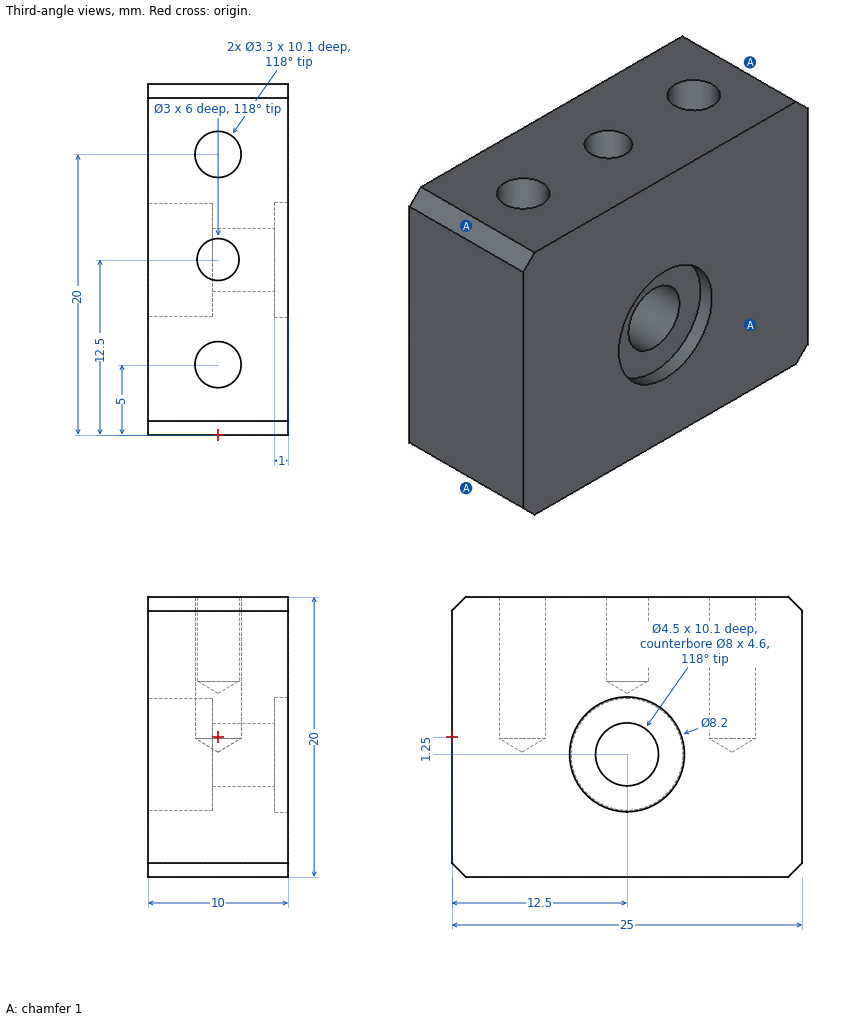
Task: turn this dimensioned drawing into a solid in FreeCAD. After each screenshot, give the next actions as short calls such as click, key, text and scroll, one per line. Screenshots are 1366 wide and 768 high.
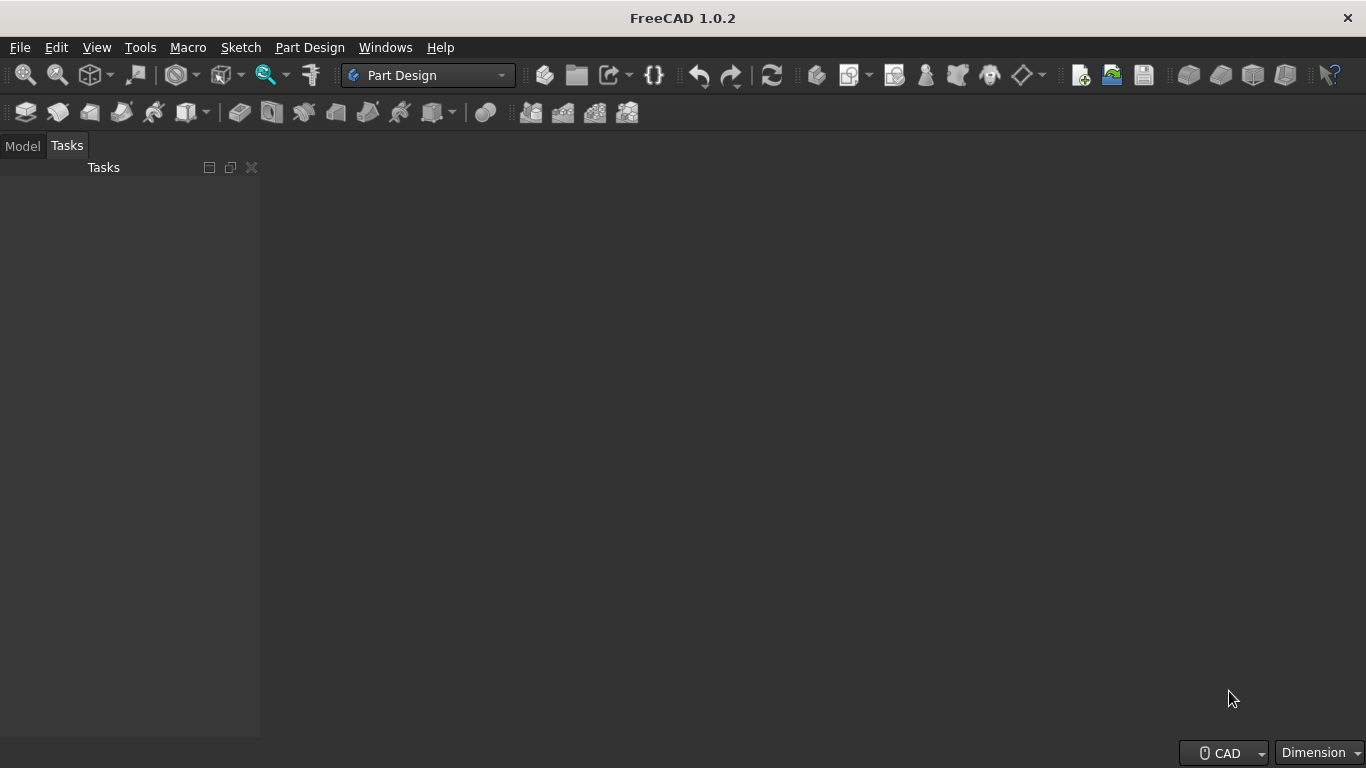
click(1080, 76)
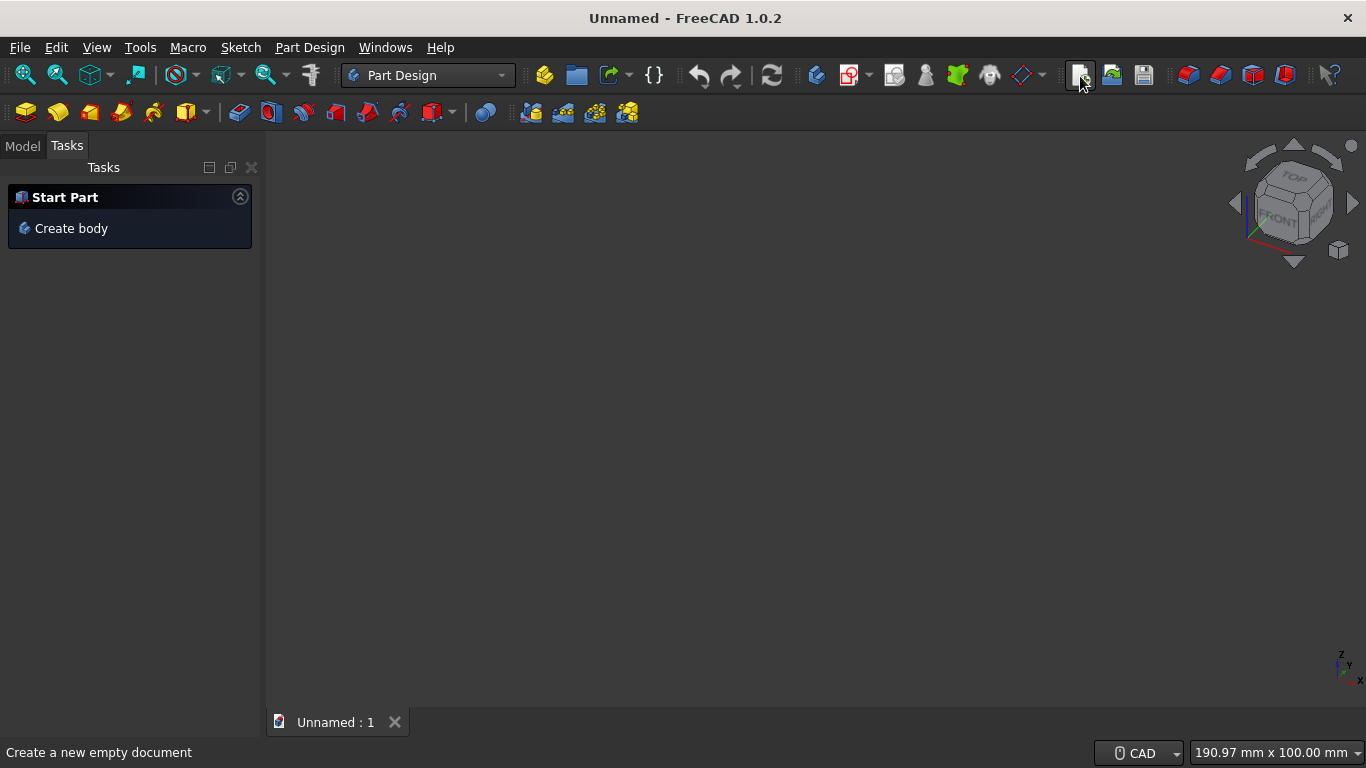
click(850, 76)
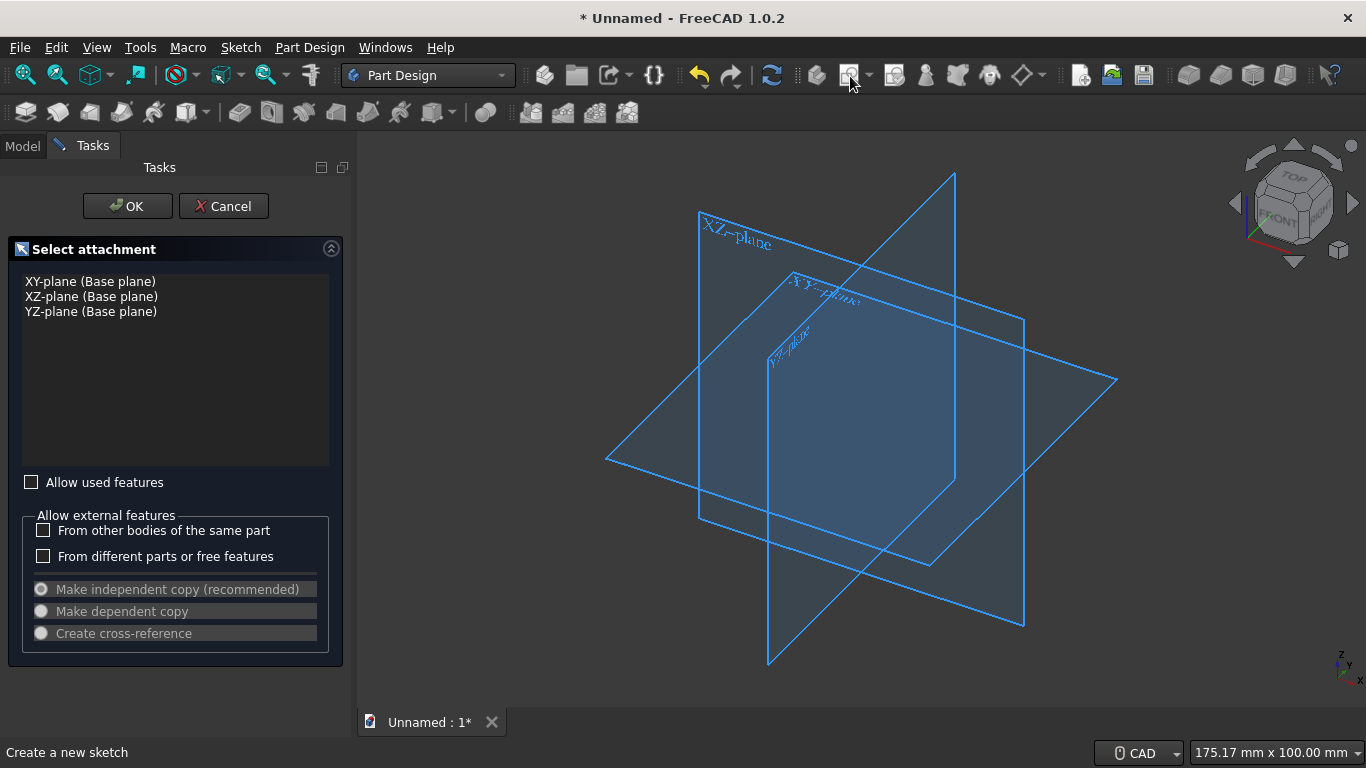
click(82, 296)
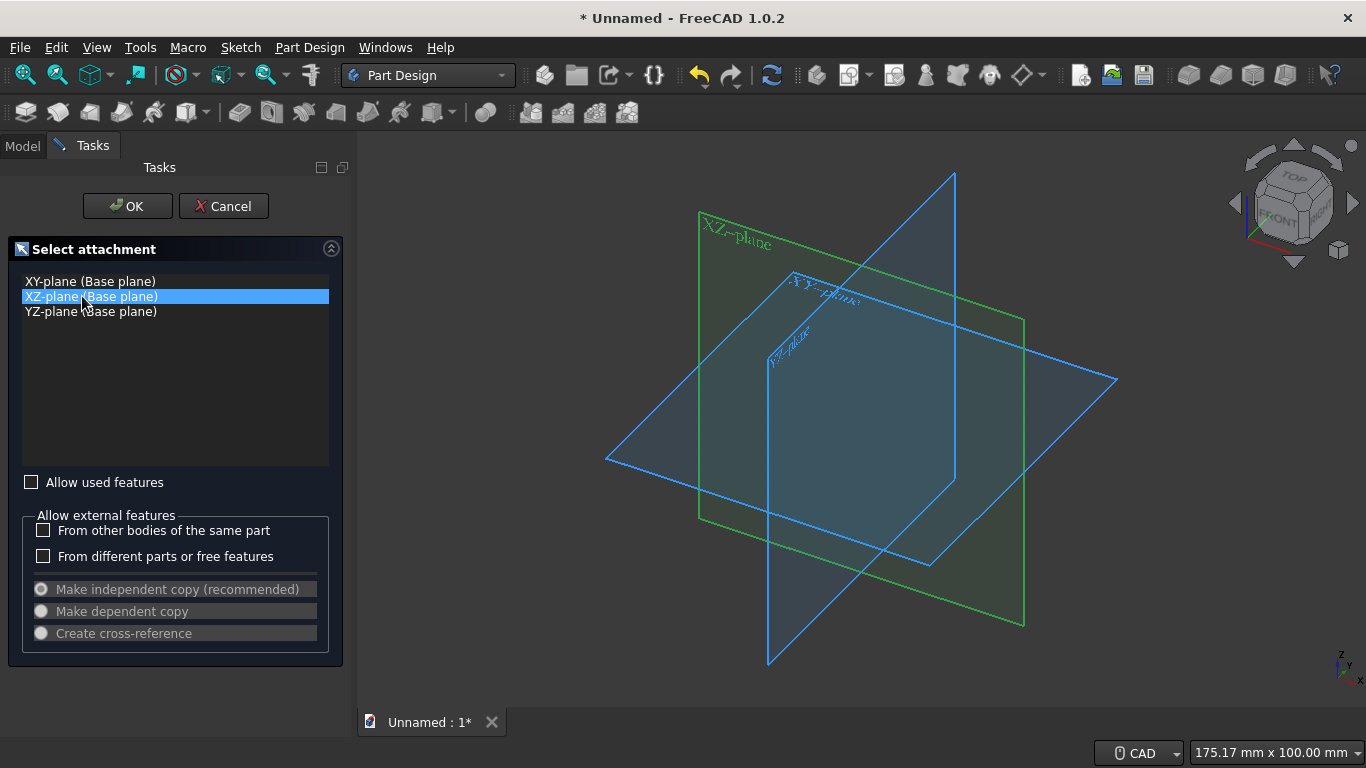
click(128, 206)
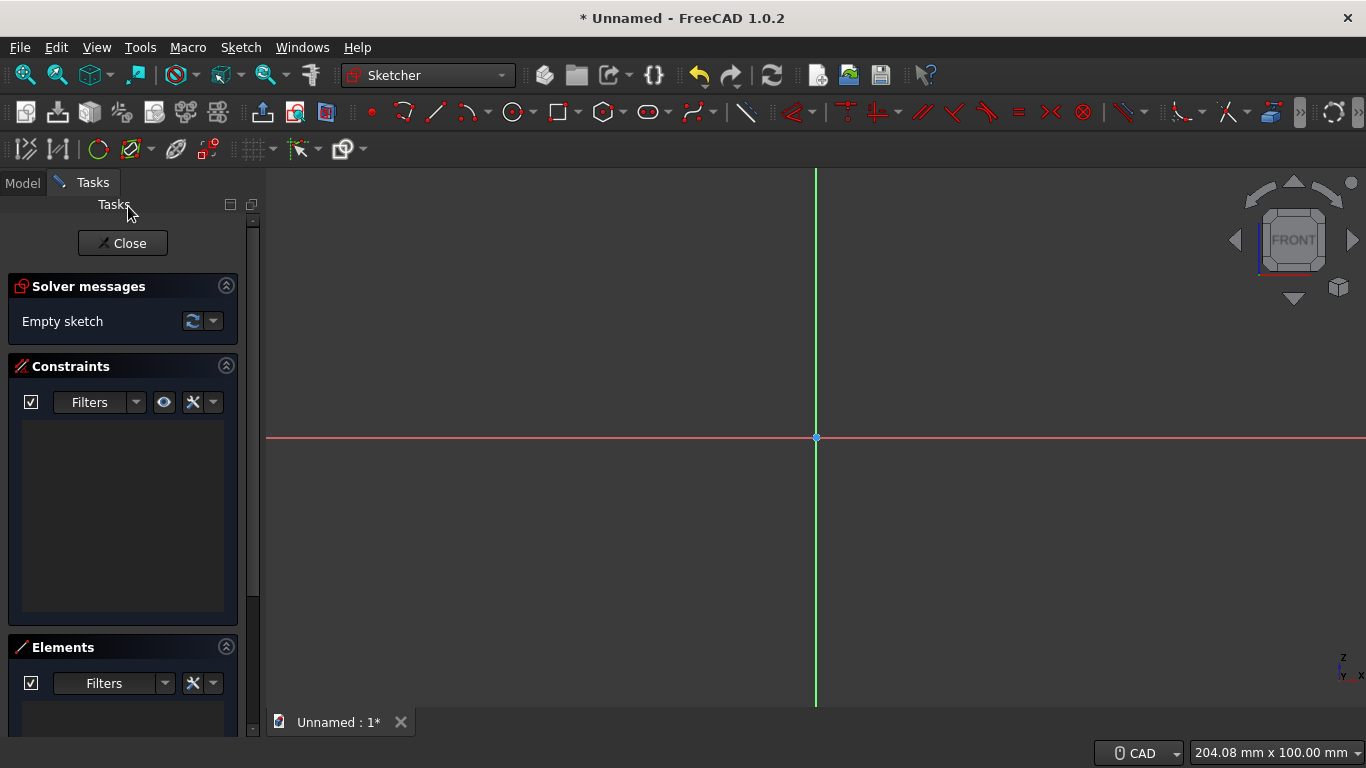
scroll(846, 438, up, 6)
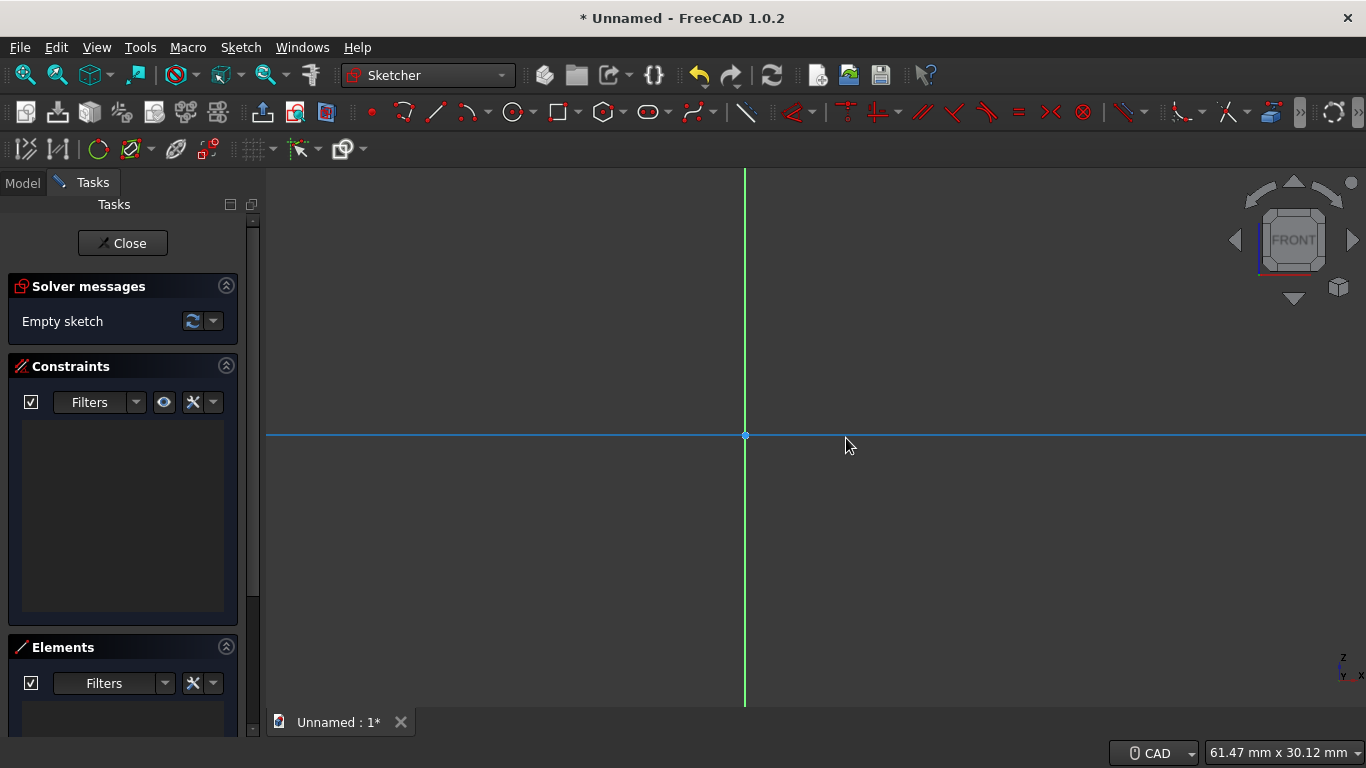
key(g)
key(v)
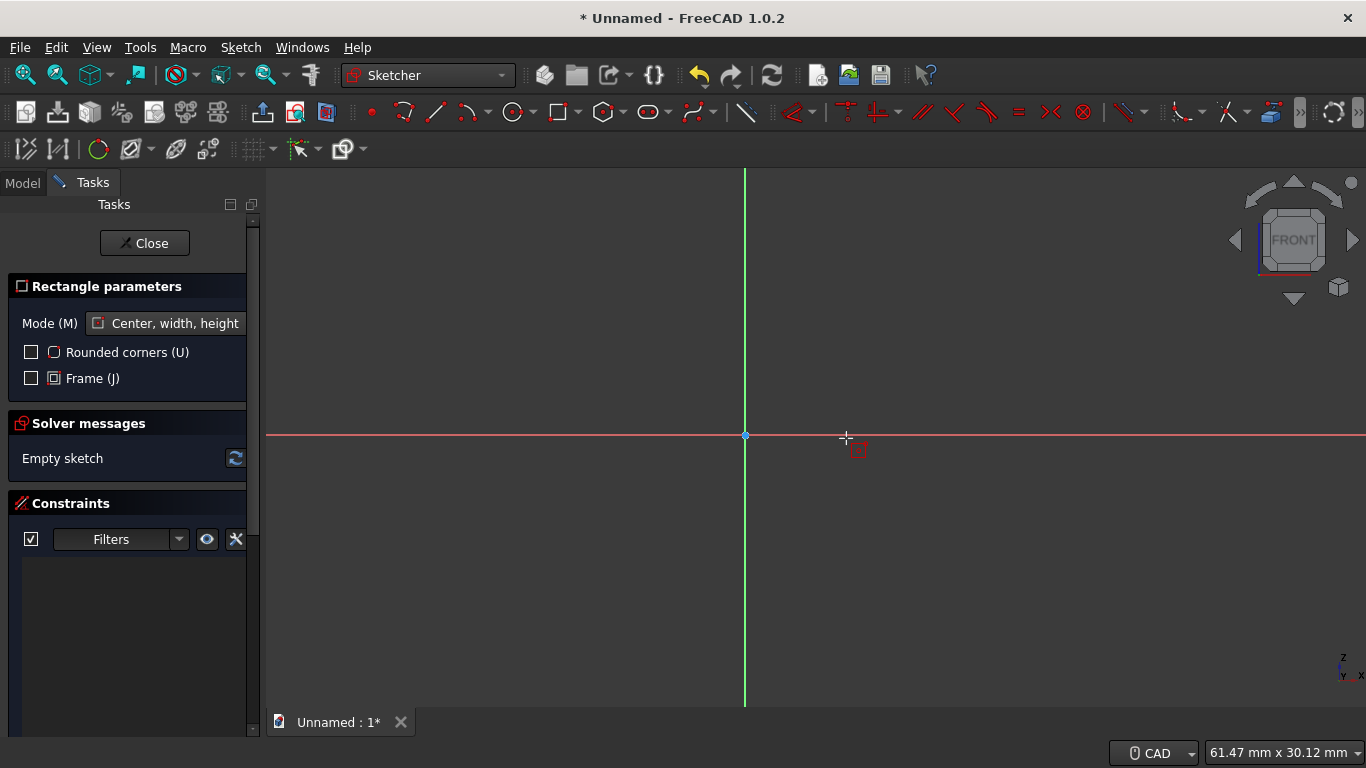
click(745, 435)
click(835, 256)
key(Escape)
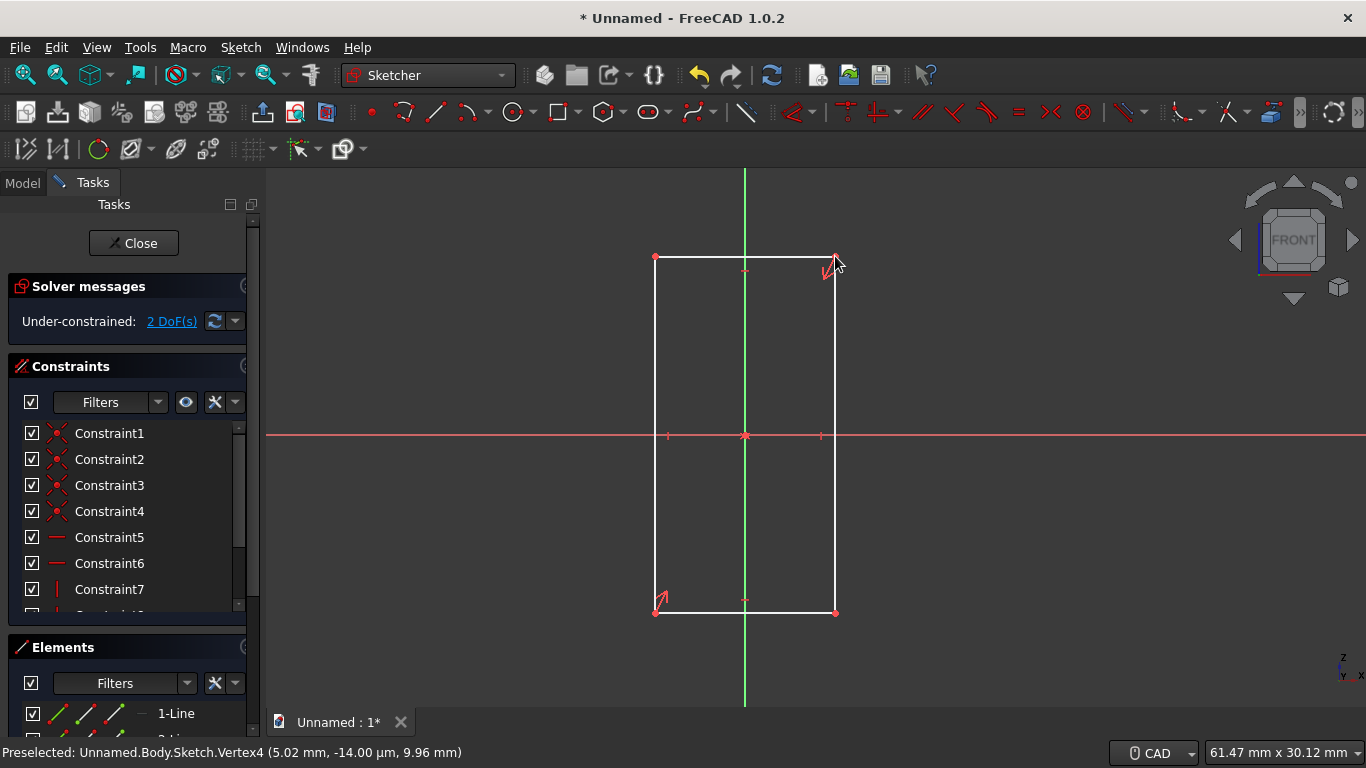
key(d)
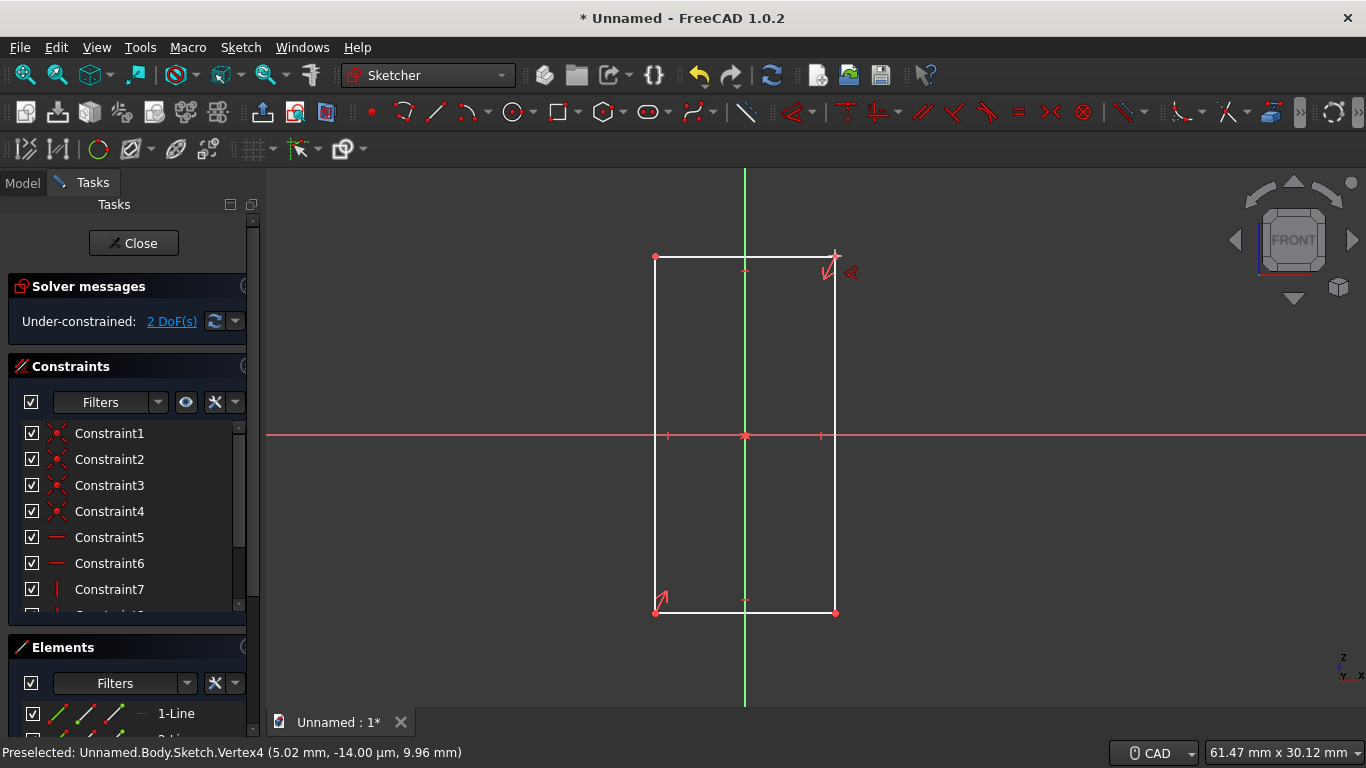
click(709, 613)
click(704, 647)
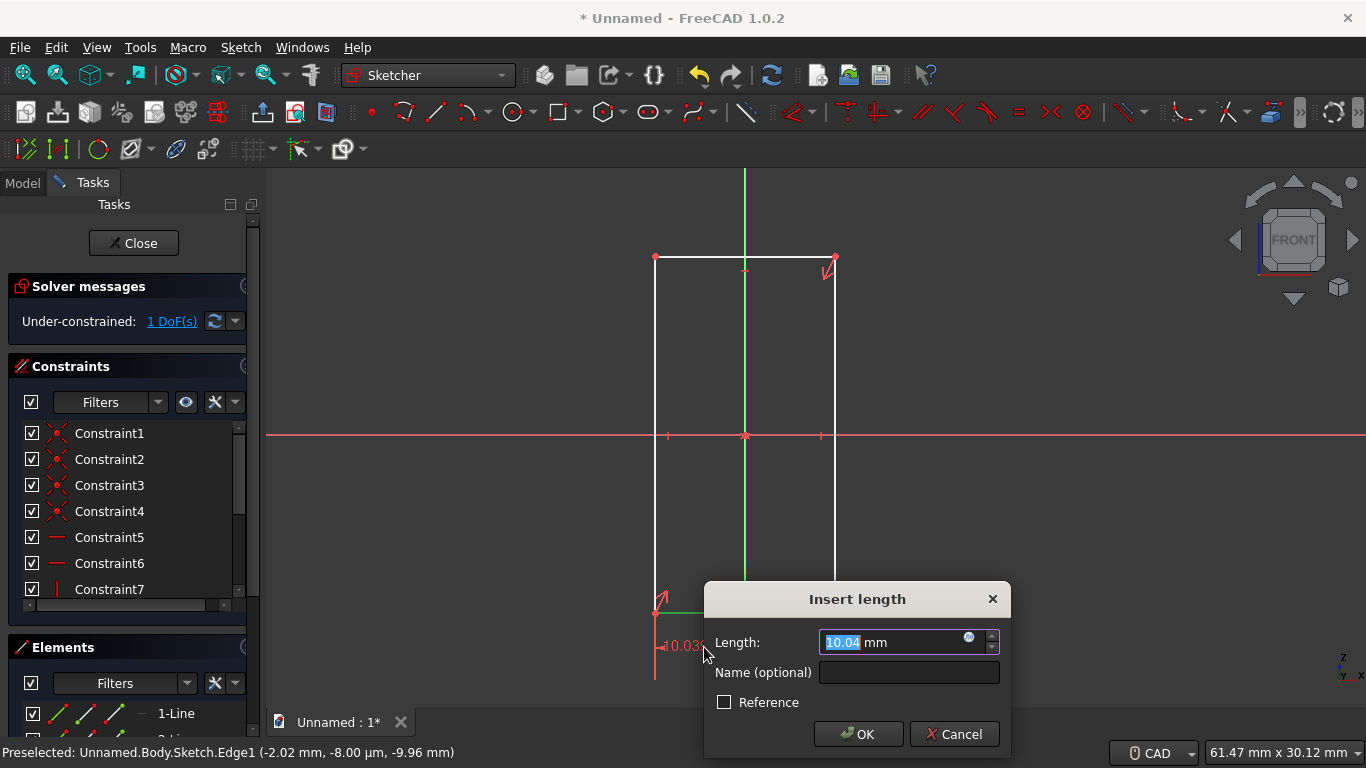
text(10)
key(Return)